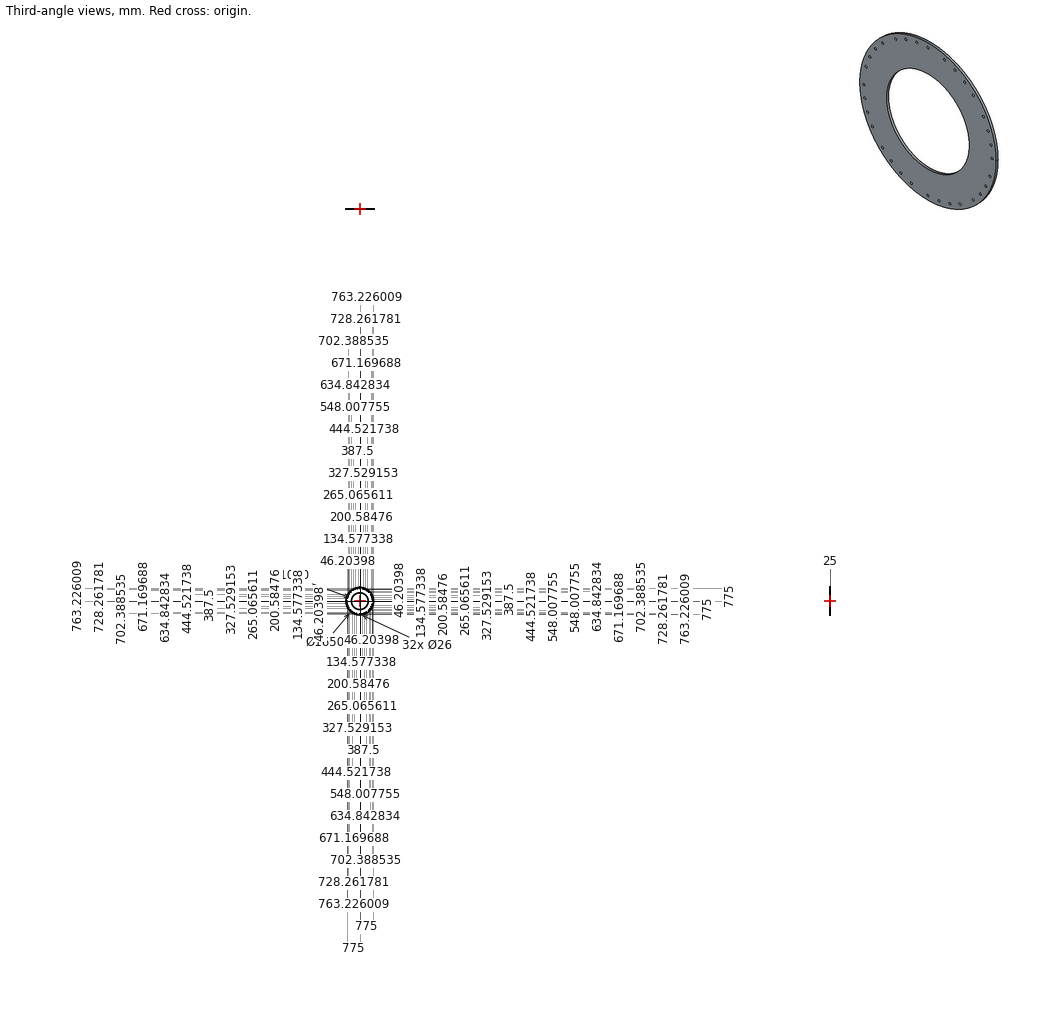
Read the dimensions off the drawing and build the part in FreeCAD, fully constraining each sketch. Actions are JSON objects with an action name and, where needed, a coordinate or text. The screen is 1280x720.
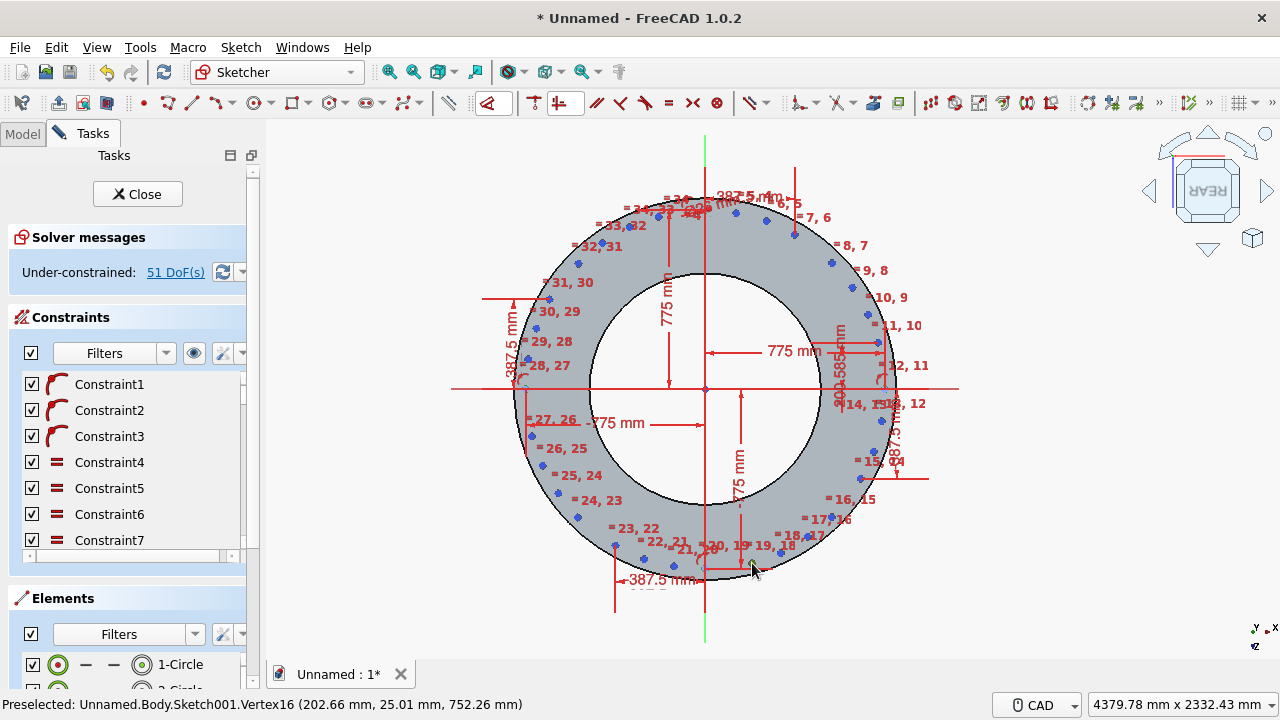
{"action": "key", "text": "l"}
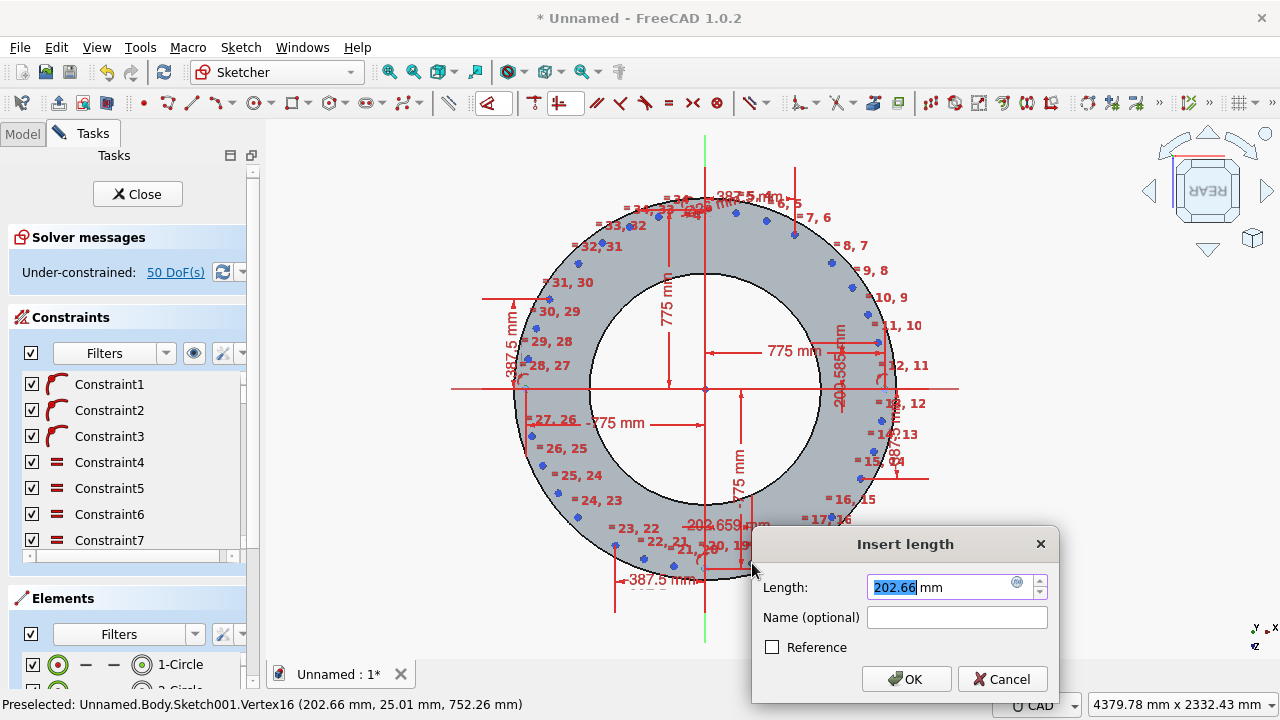
{"action": "type", "text": "200.58476"}
{"action": "key", "text": "Return"}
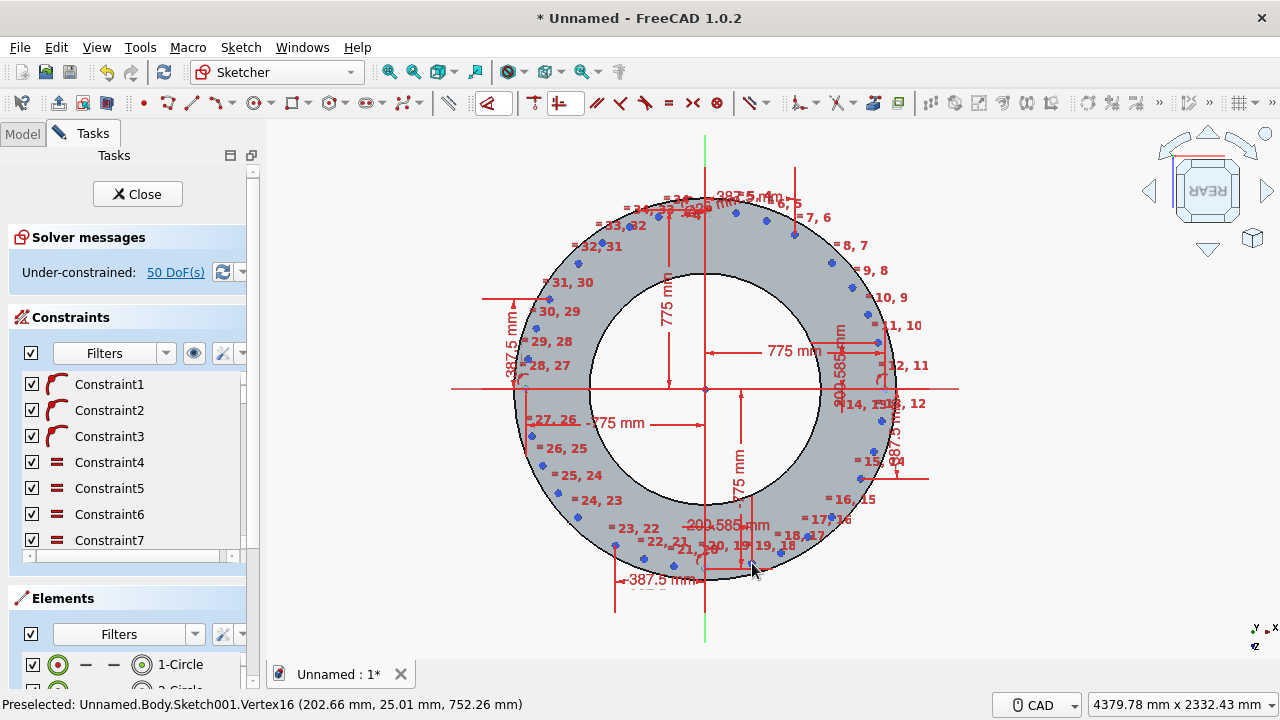
{"action": "left_click", "coordinate": [532, 436]}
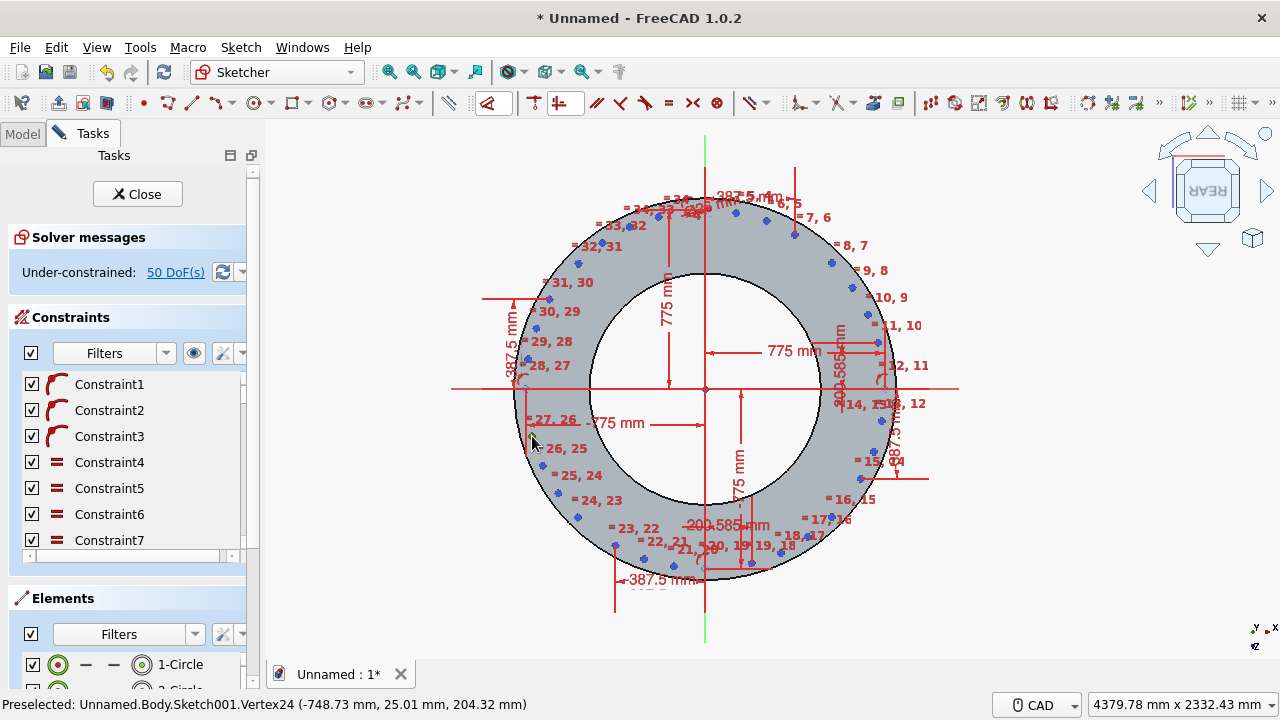
{"action": "key", "text": "i"}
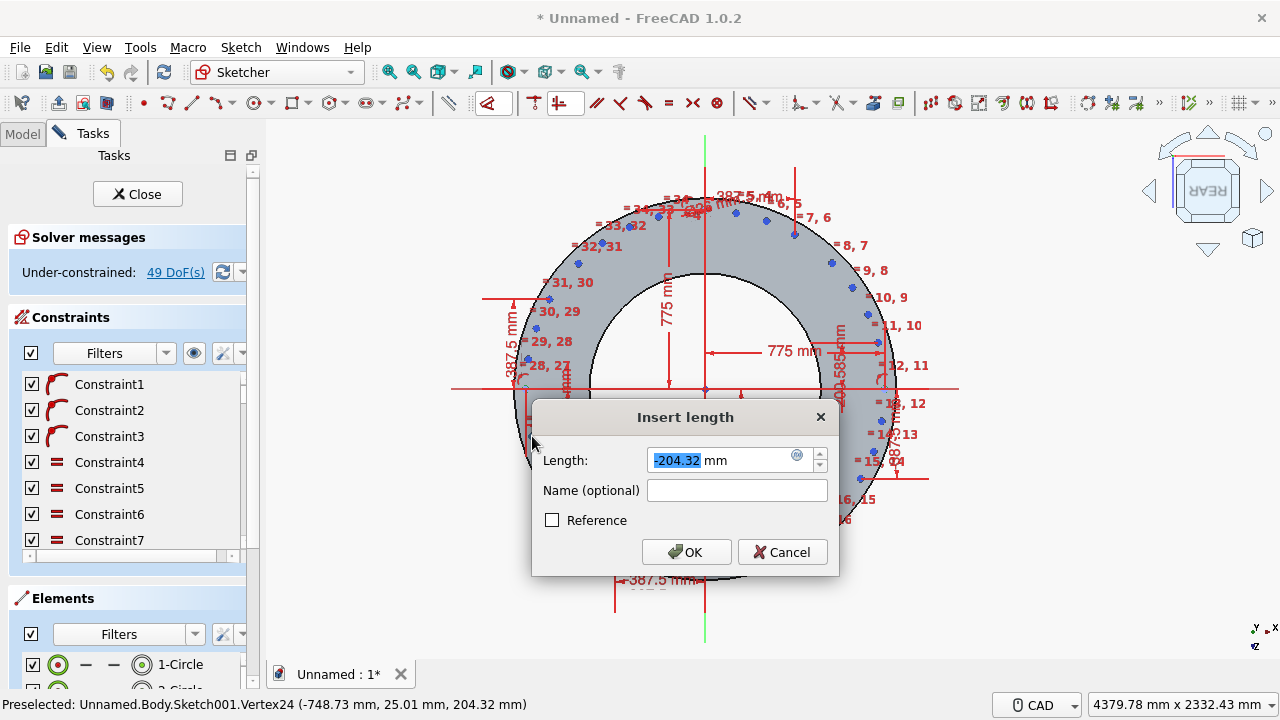
{"action": "type", "text": "-200.58476"}
{"action": "key", "text": "Return"}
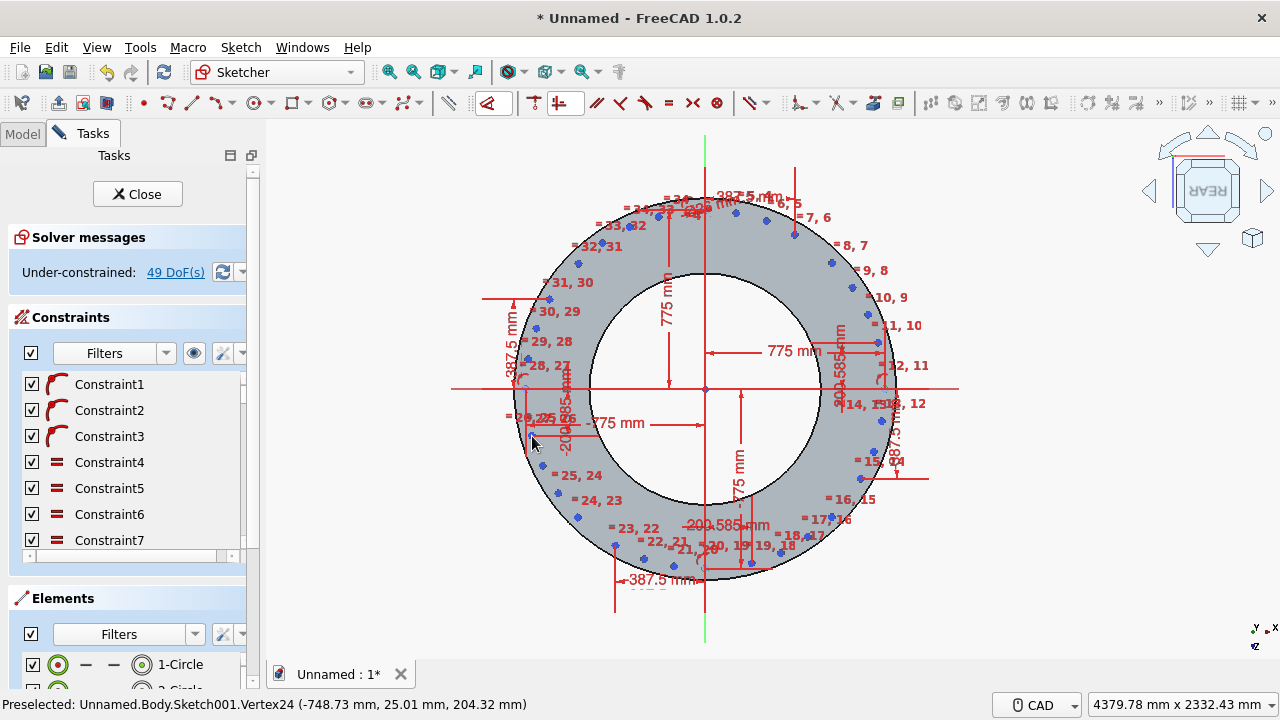
{"action": "left_click", "coordinate": [659, 217]}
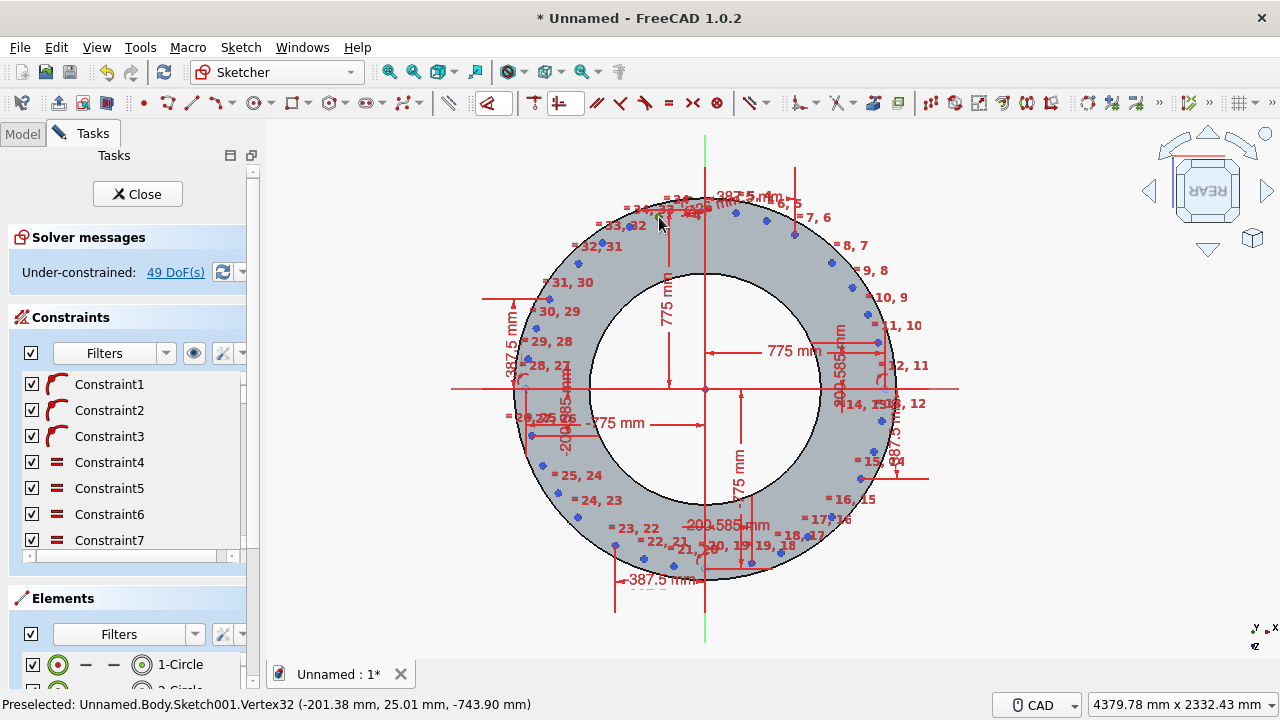
{"action": "key", "text": "l"}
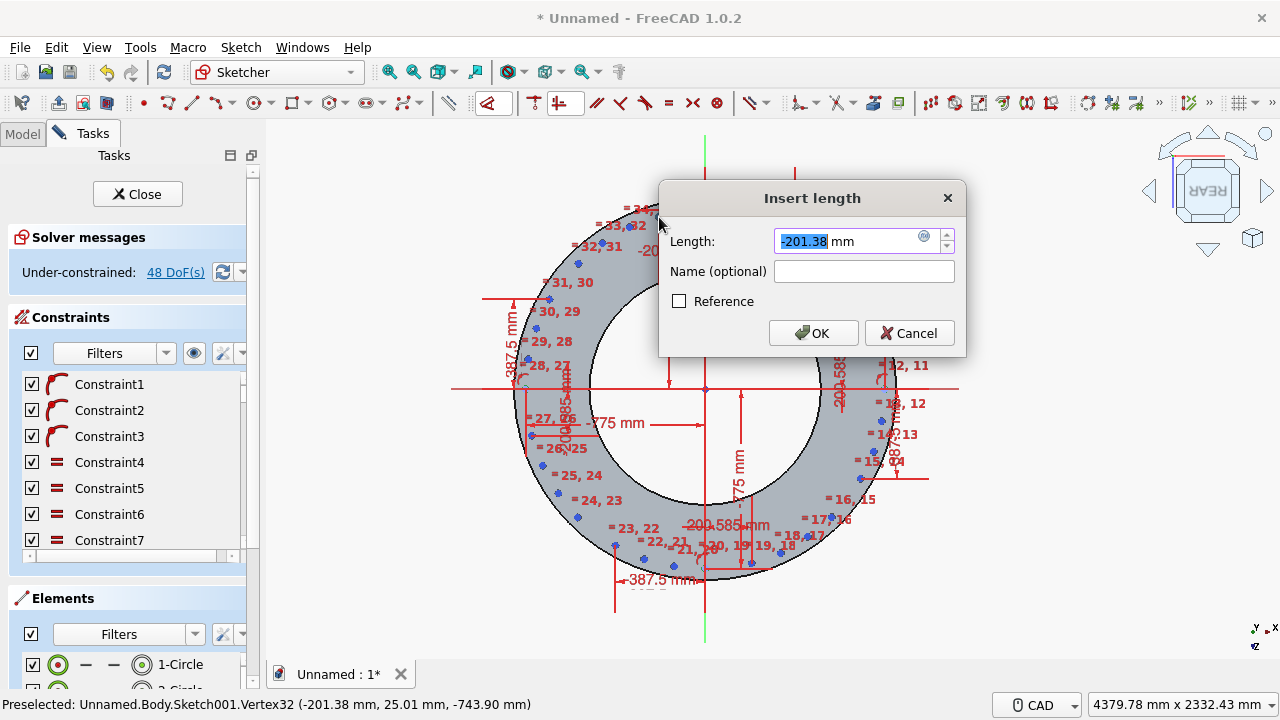
{"action": "type", "text": "-200.58476"}
{"action": "key", "text": "Return"}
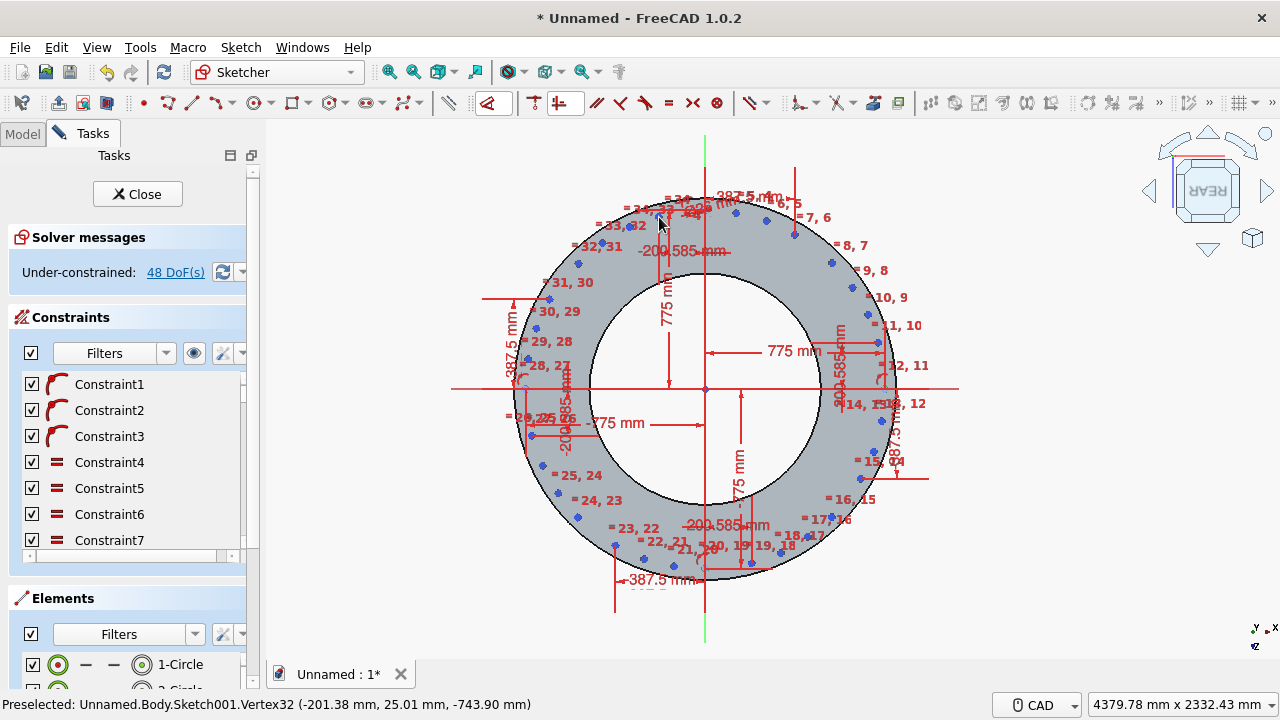
{"action": "scroll", "coordinate": [868, 315], "scroll_direction": "up", "scroll_amount": 7}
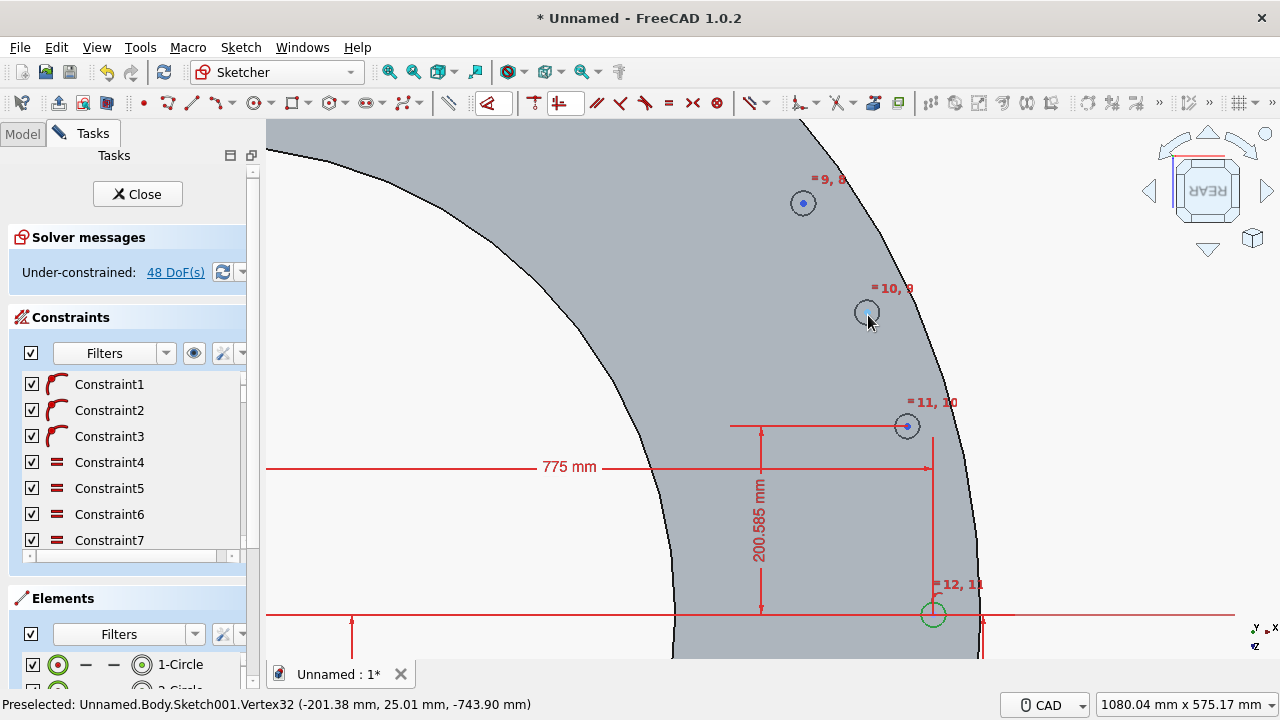
{"action": "left_click", "coordinate": [867, 313]}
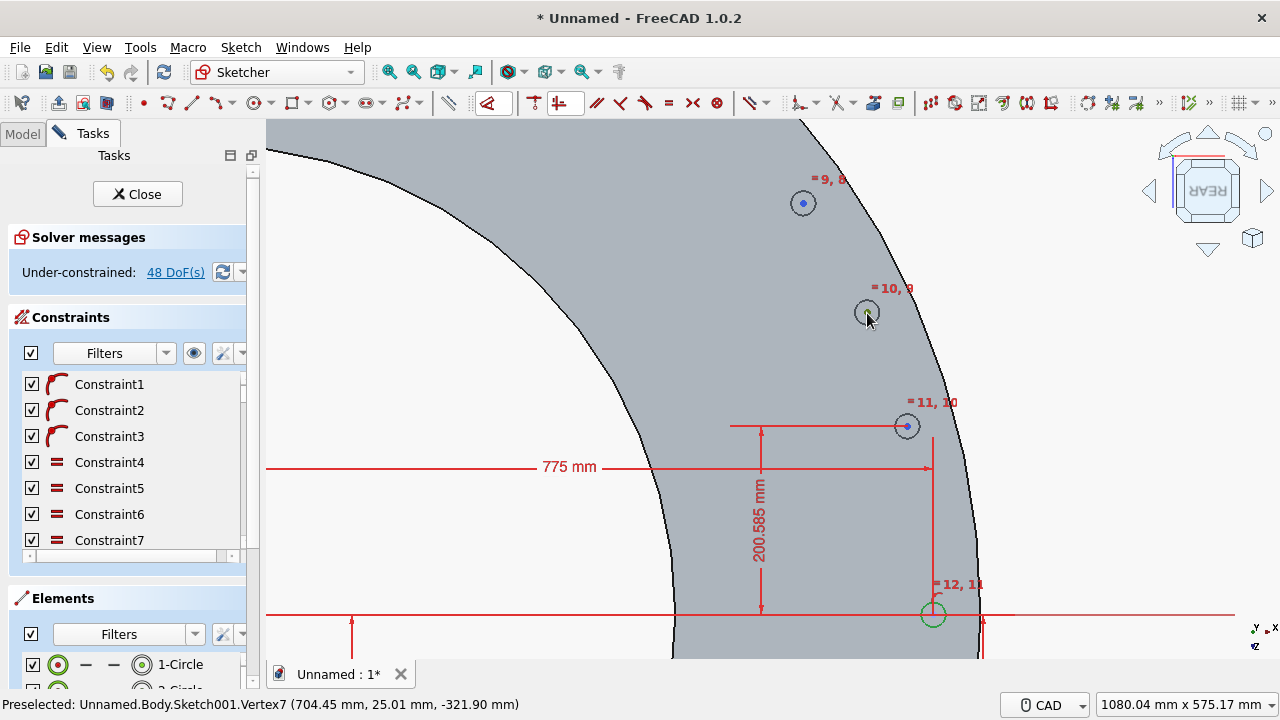
{"action": "left_click", "coordinate": [907, 426]}